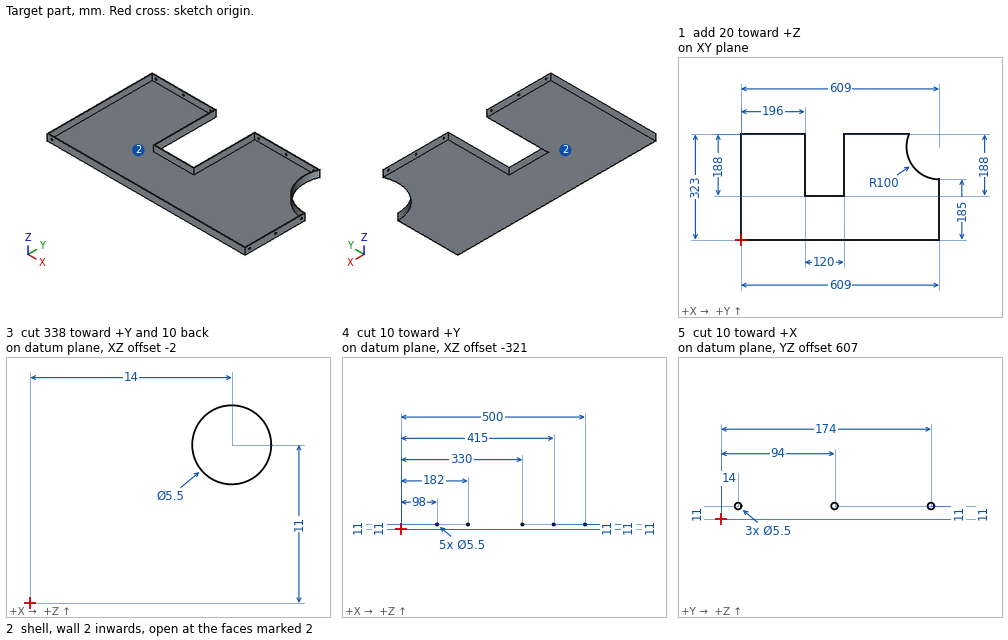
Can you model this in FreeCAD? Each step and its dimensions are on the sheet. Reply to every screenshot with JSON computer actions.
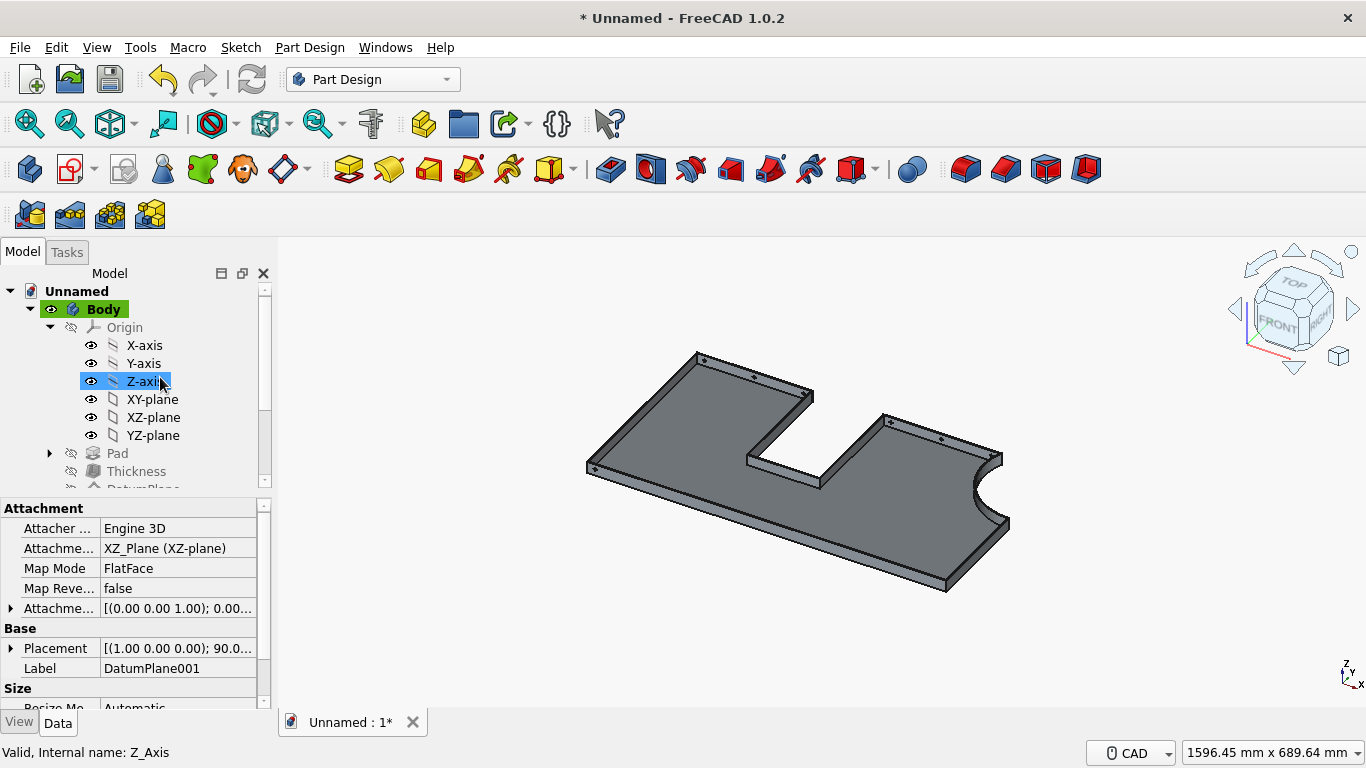
{"action": "left_click", "coordinate": [136, 435]}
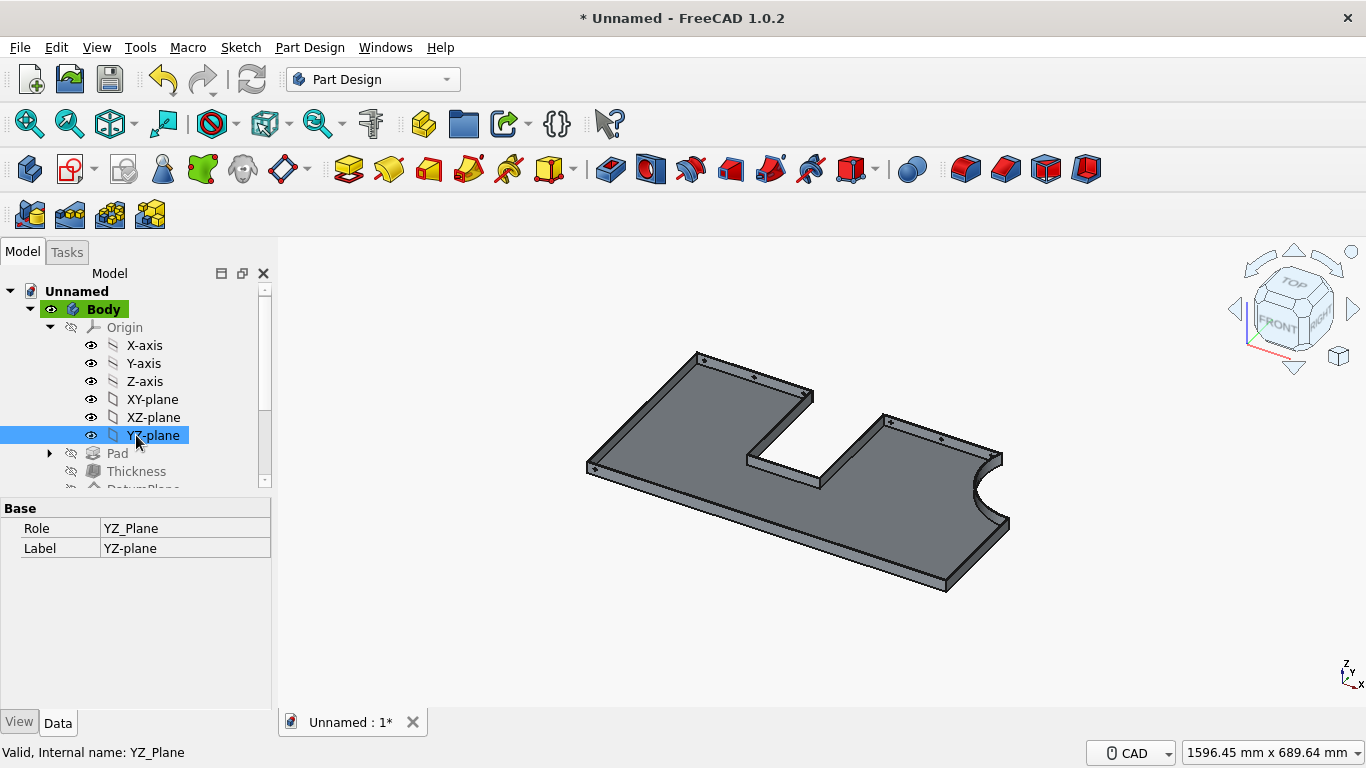
{"action": "left_click", "coordinate": [284, 170]}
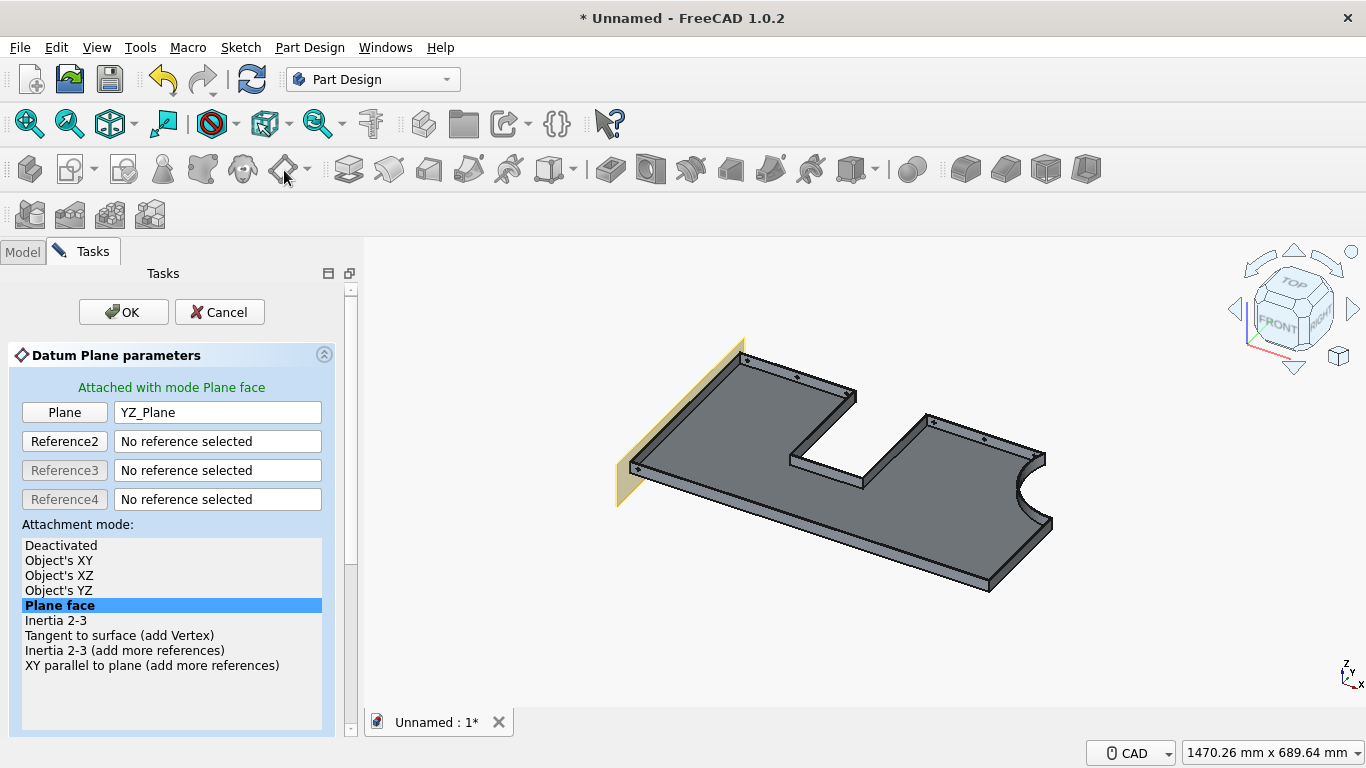
{"action": "scroll", "coordinate": [351, 510], "scroll_direction": "down", "scroll_amount": 3}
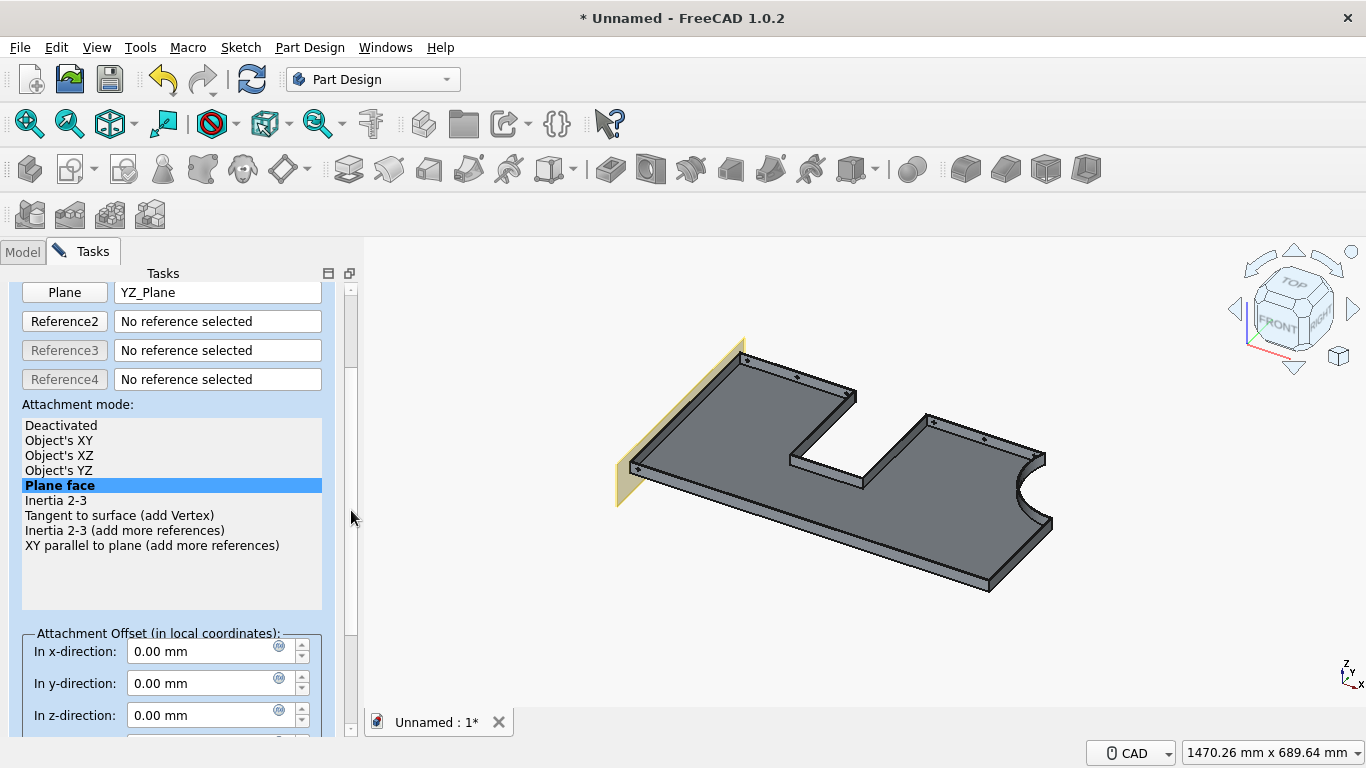
{"action": "triple_click", "coordinate": [210, 655]}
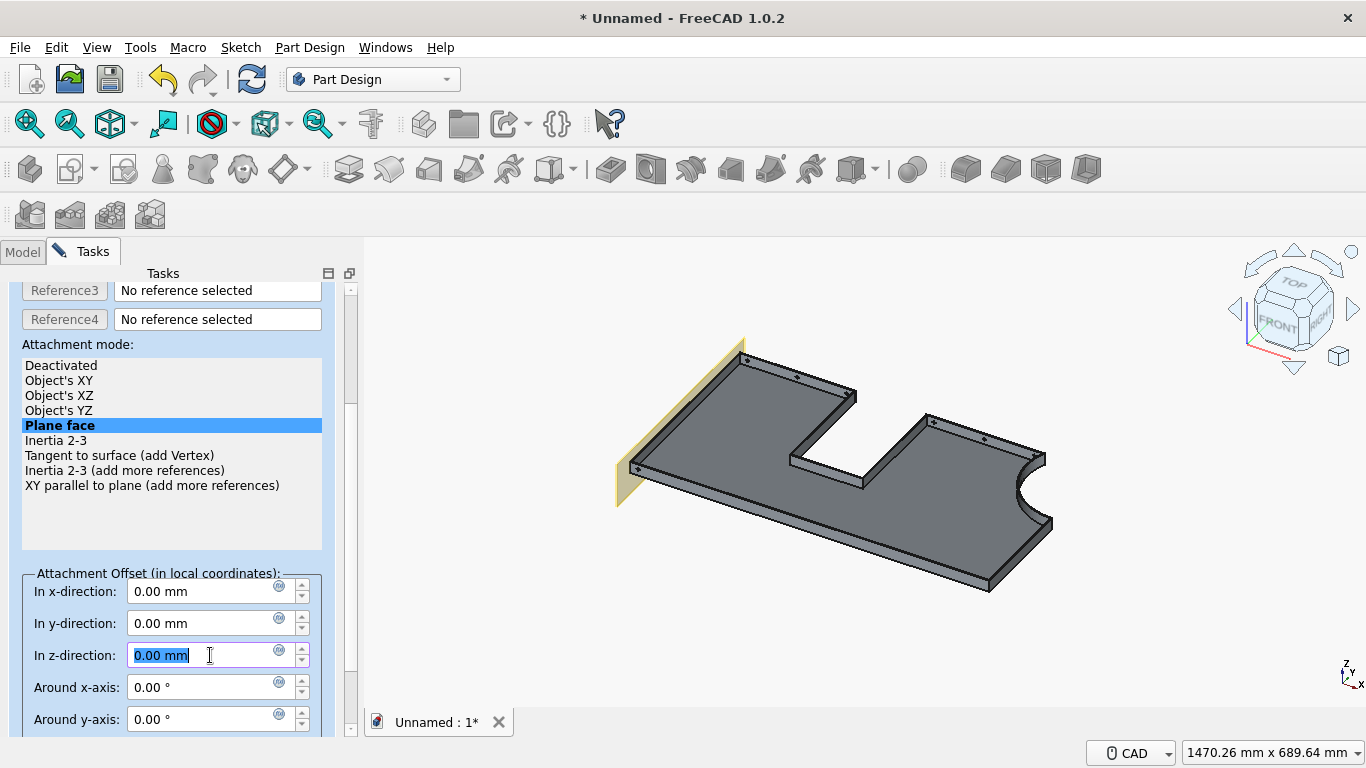
{"action": "type", "text": "607"}
{"action": "key", "text": "Tab"}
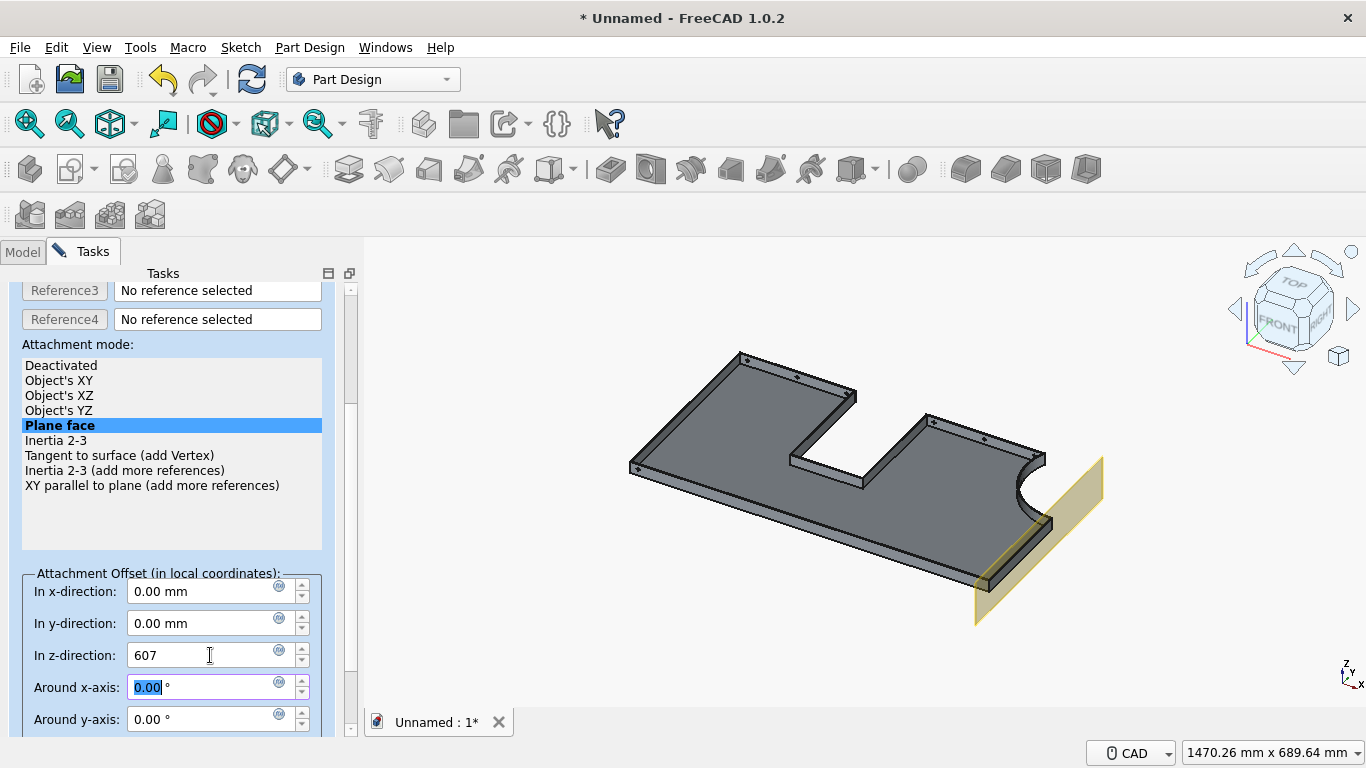
{"action": "scroll", "coordinate": [351, 510], "scroll_direction": "up", "scroll_amount": 4}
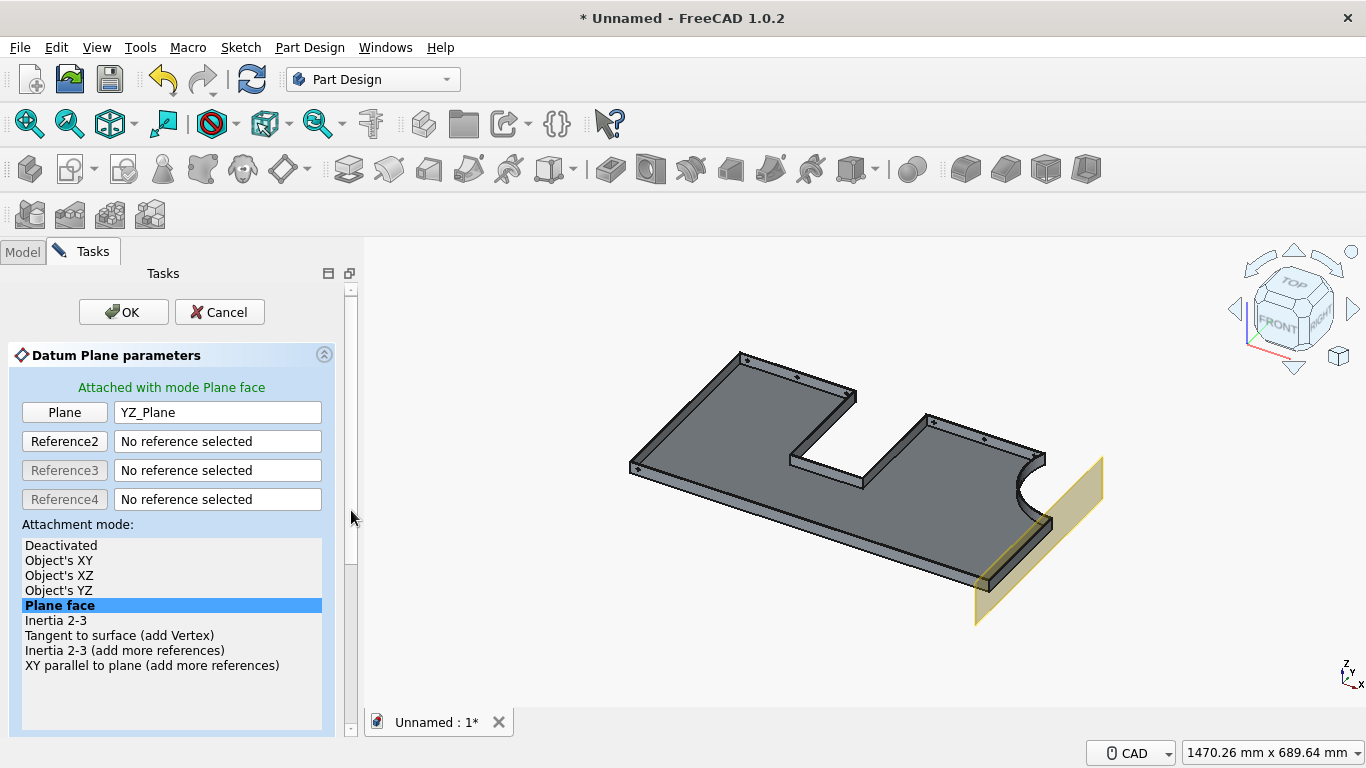
{"action": "left_click", "coordinate": [124, 312]}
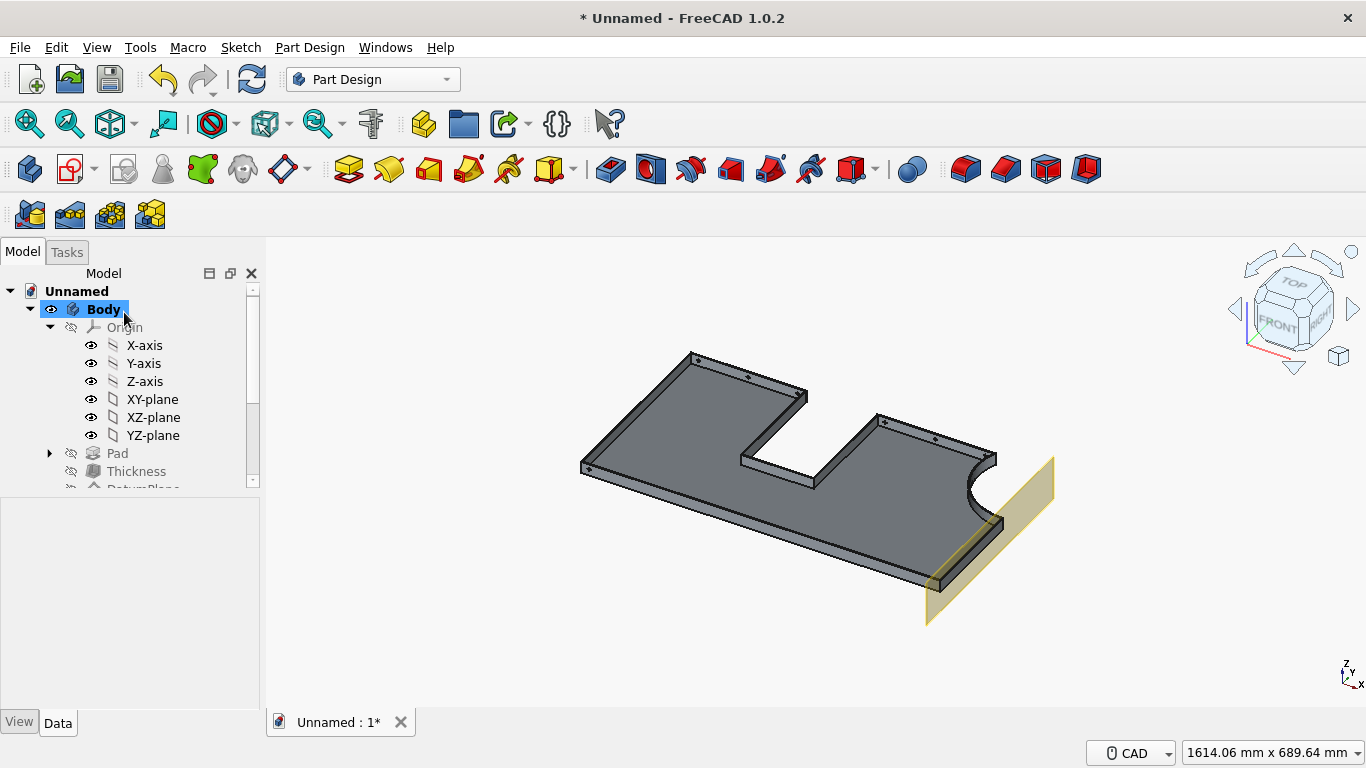
{"action": "scroll", "coordinate": [100, 377], "scroll_direction": "down", "scroll_amount": 3}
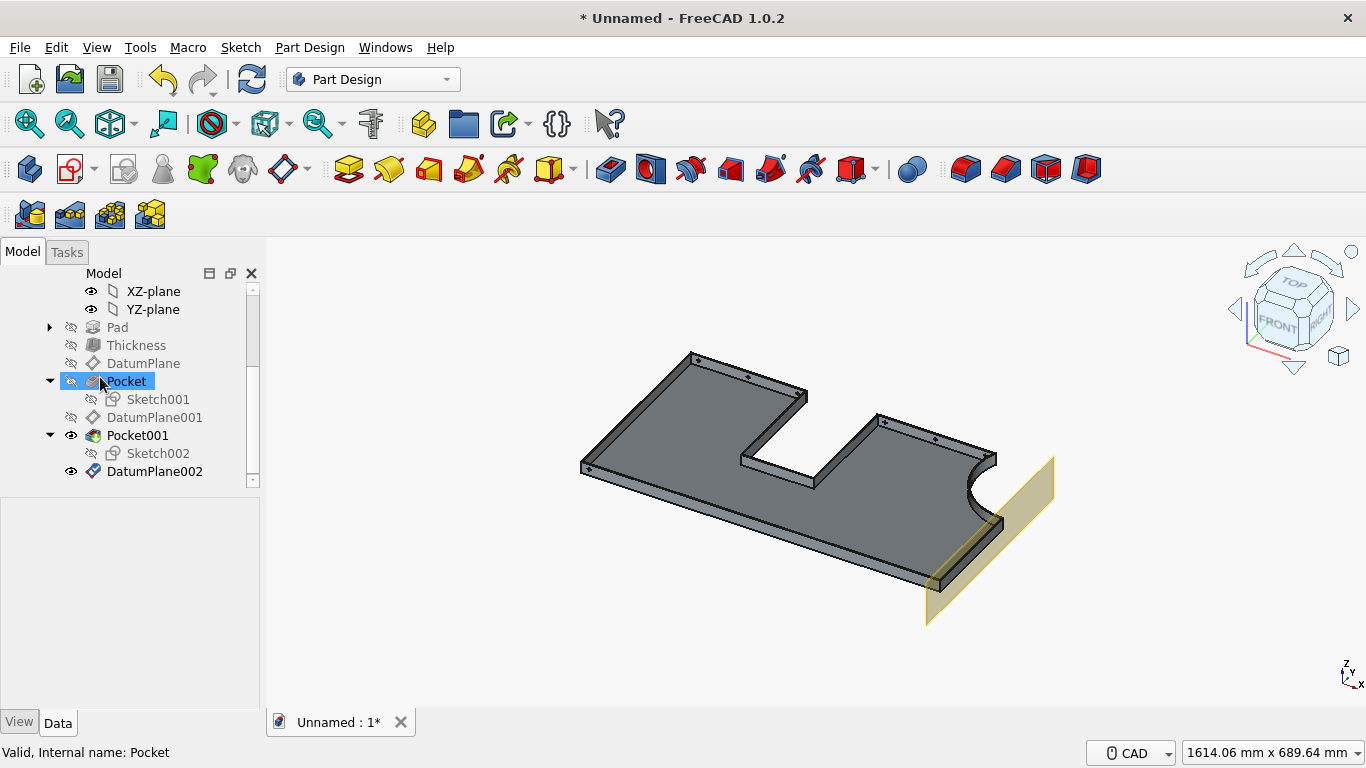
{"action": "left_click", "coordinate": [116, 471]}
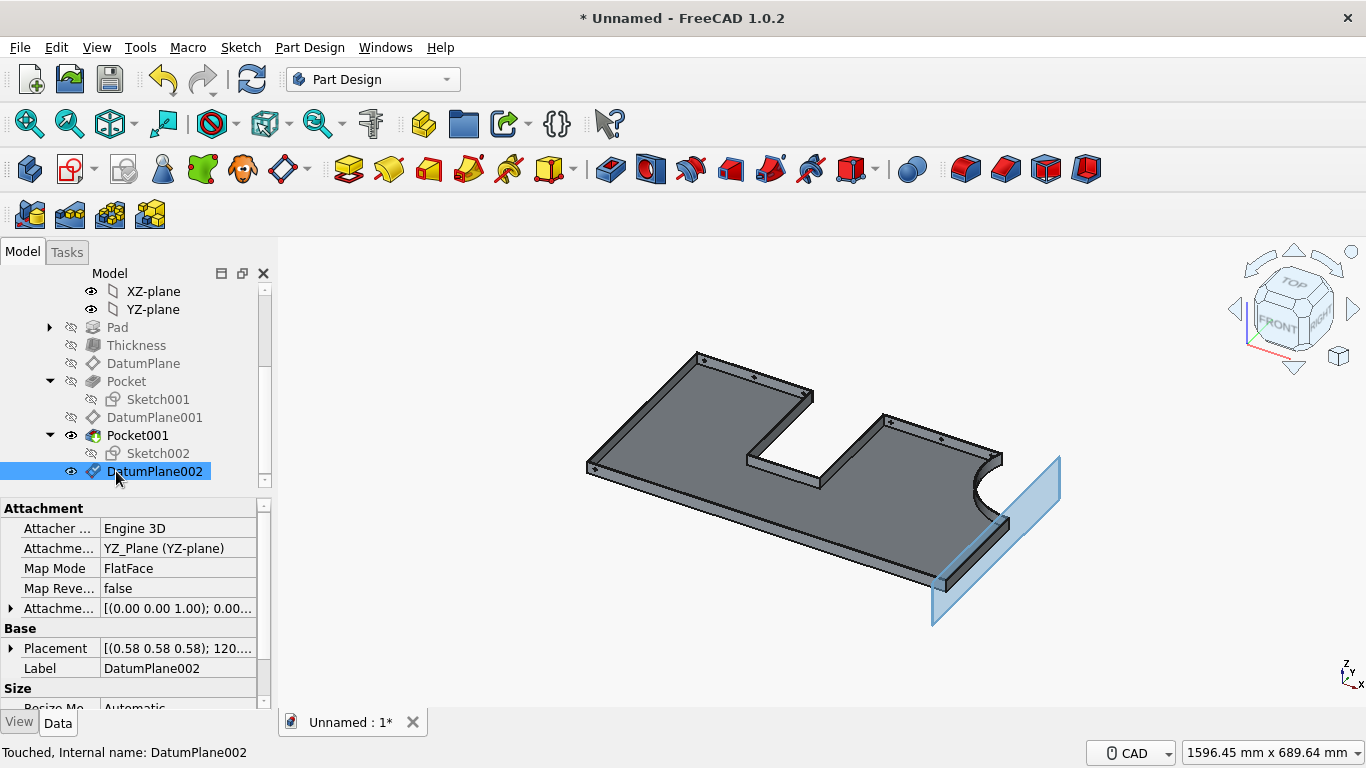
{"action": "left_click", "coordinate": [70, 170]}